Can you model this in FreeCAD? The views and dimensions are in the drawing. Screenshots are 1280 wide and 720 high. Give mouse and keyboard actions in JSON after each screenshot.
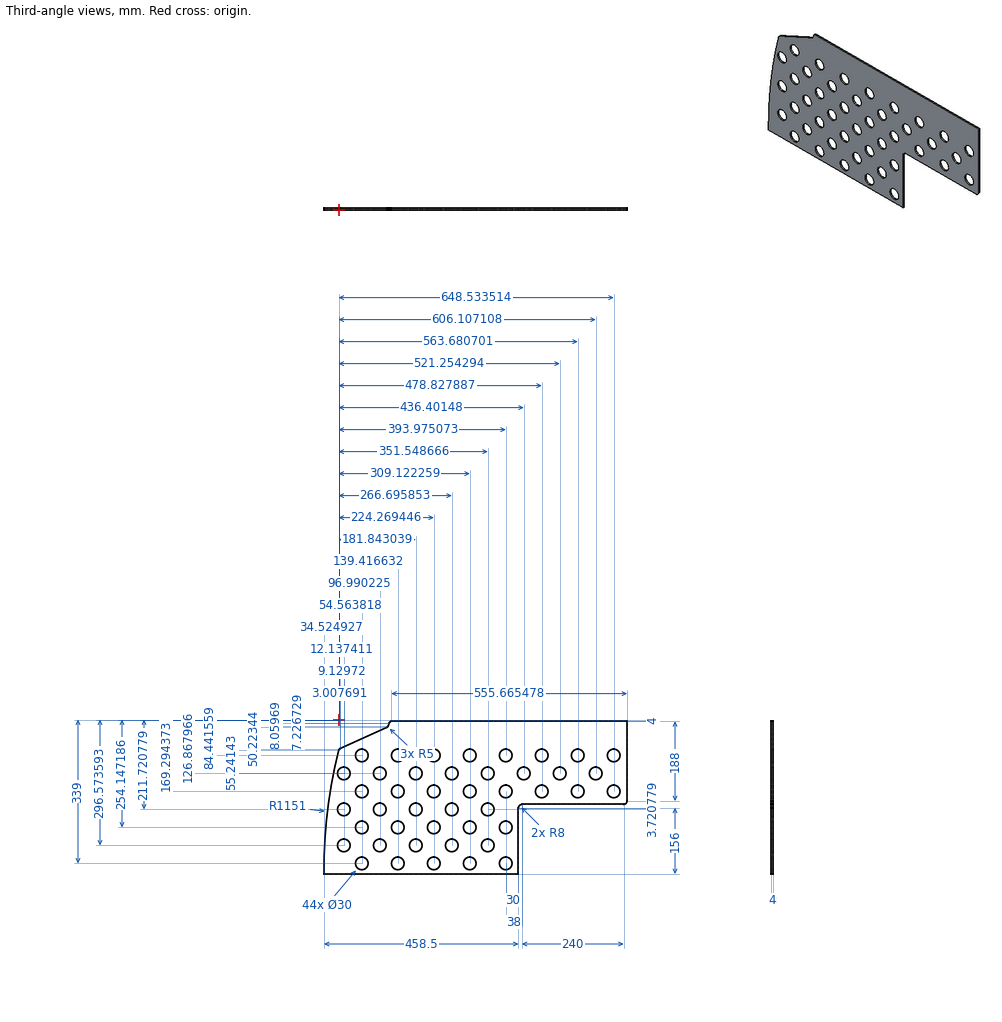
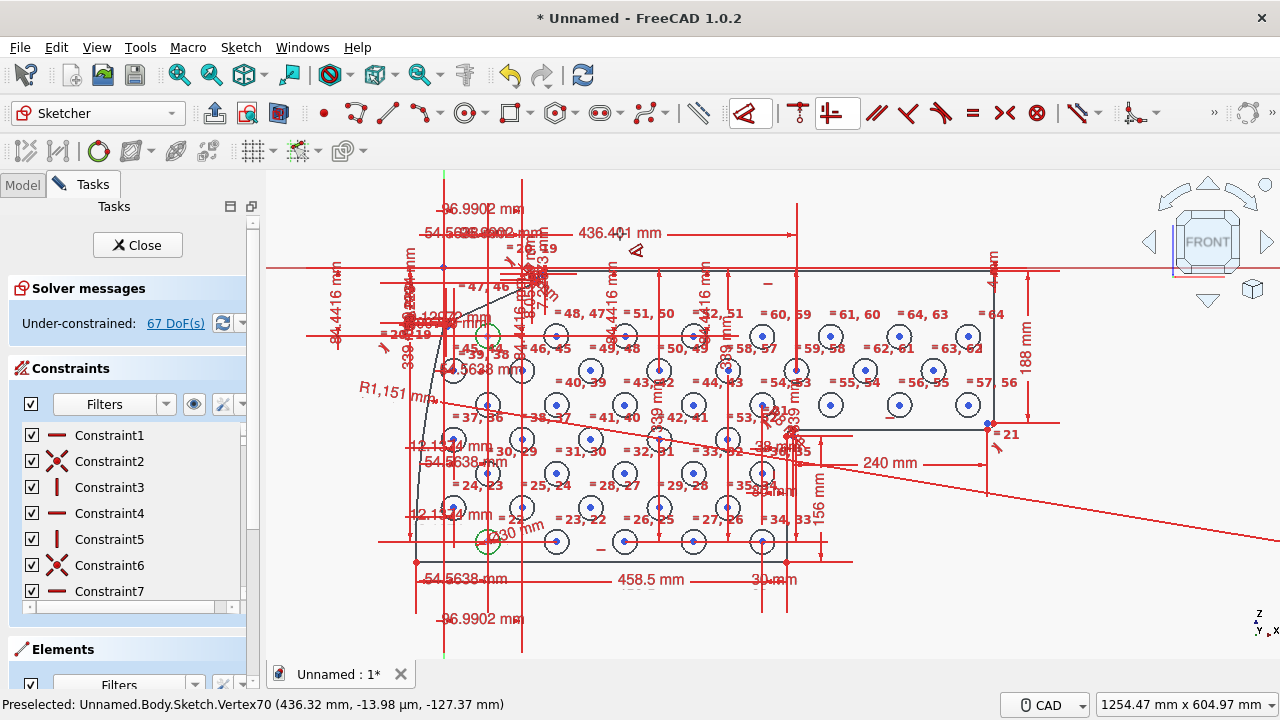
{"action": "left_click", "coordinate": [762, 337]}
{"action": "left_click", "coordinate": [796, 302]}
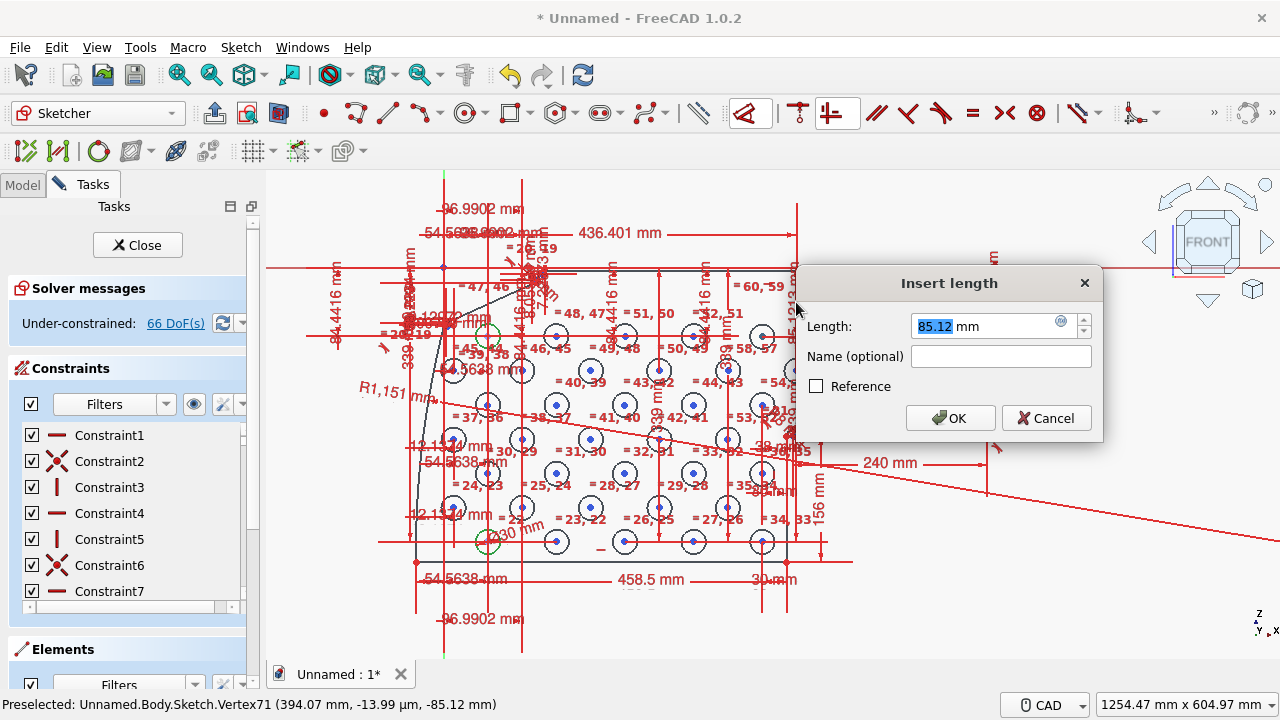
{"action": "type", "text": "84.441559"}
{"action": "key", "text": "Return"}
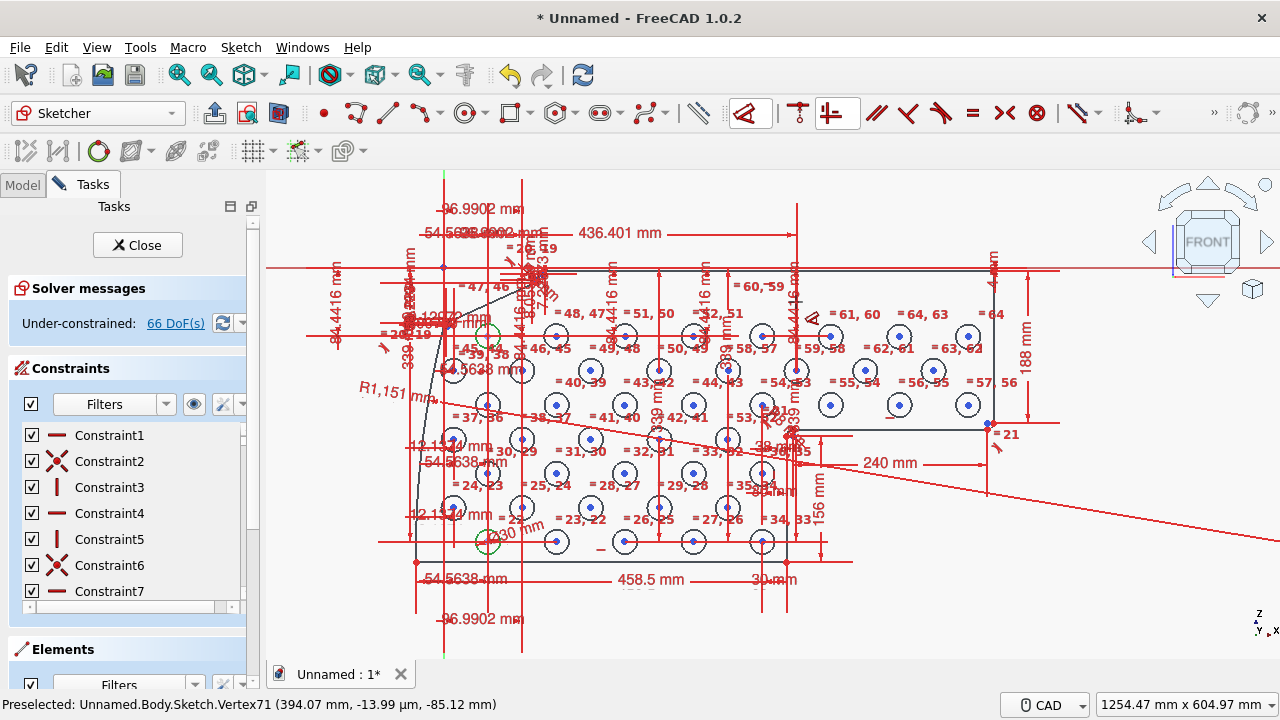
{"action": "left_click", "coordinate": [831, 337]}
{"action": "left_click", "coordinate": [865, 326]}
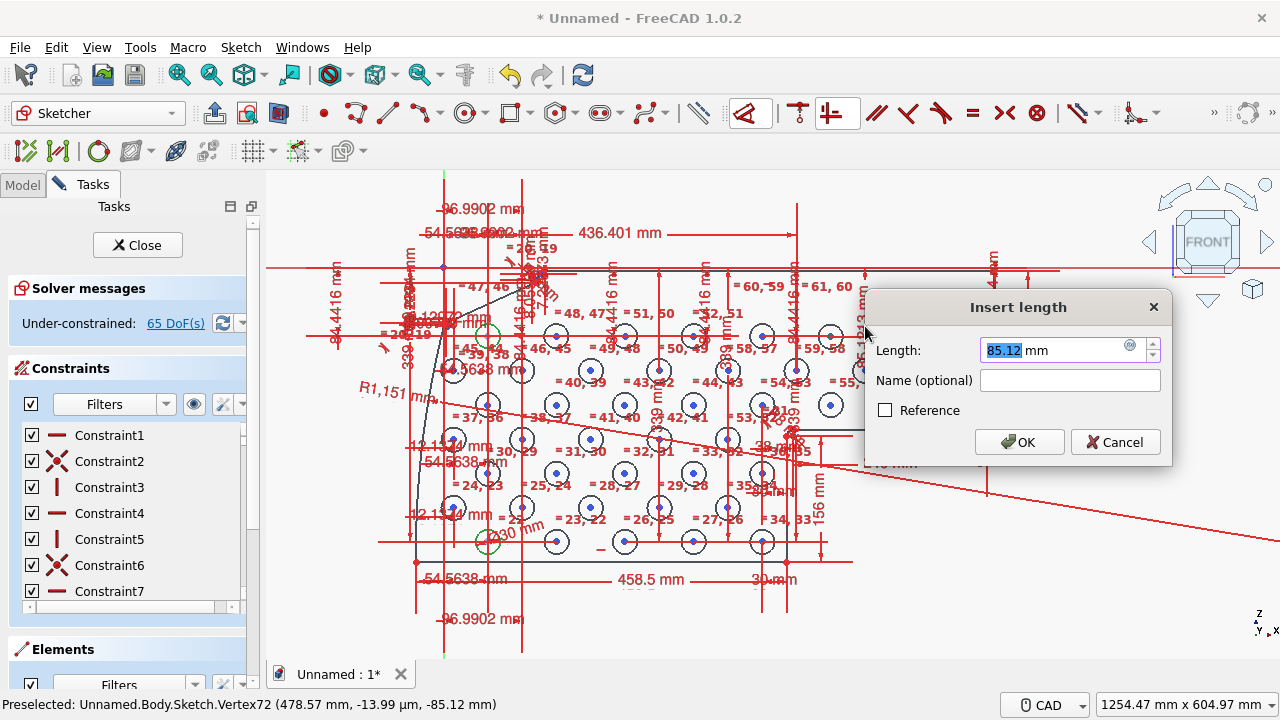
{"action": "type", "text": "84.441559"}
{"action": "key", "text": "Return"}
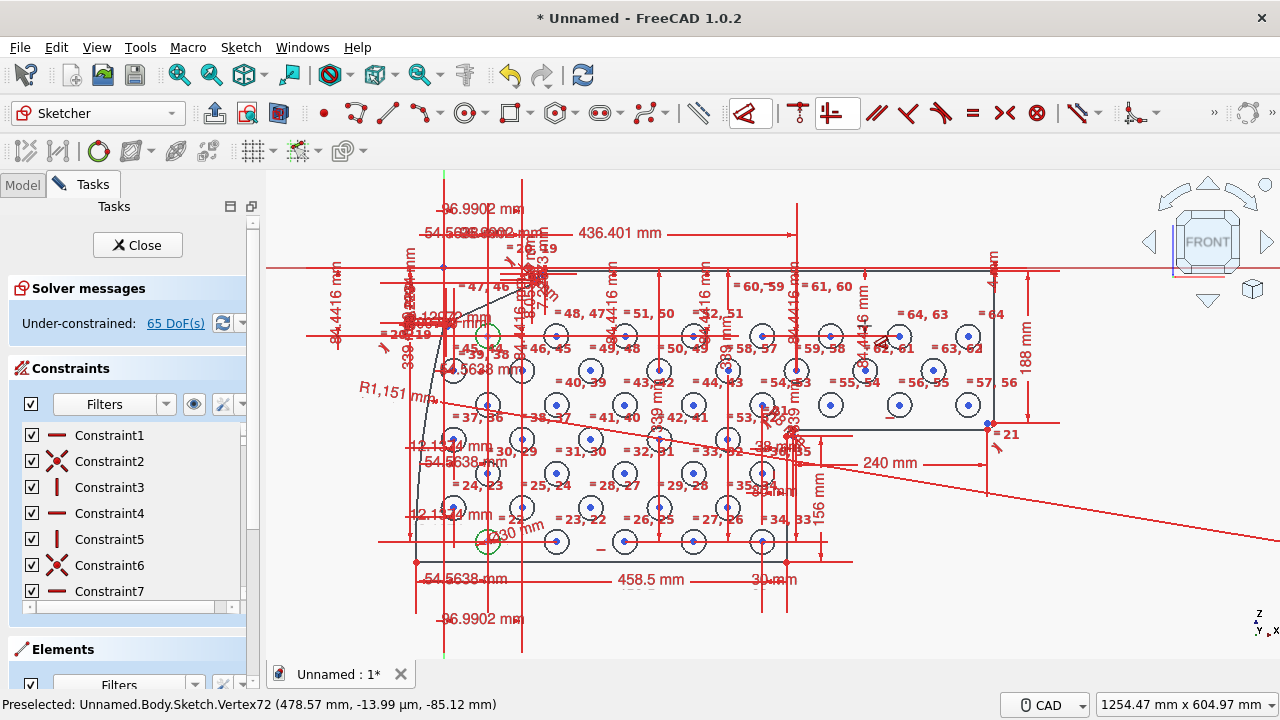
{"action": "left_click", "coordinate": [899, 337]}
{"action": "left_click", "coordinate": [933, 302]}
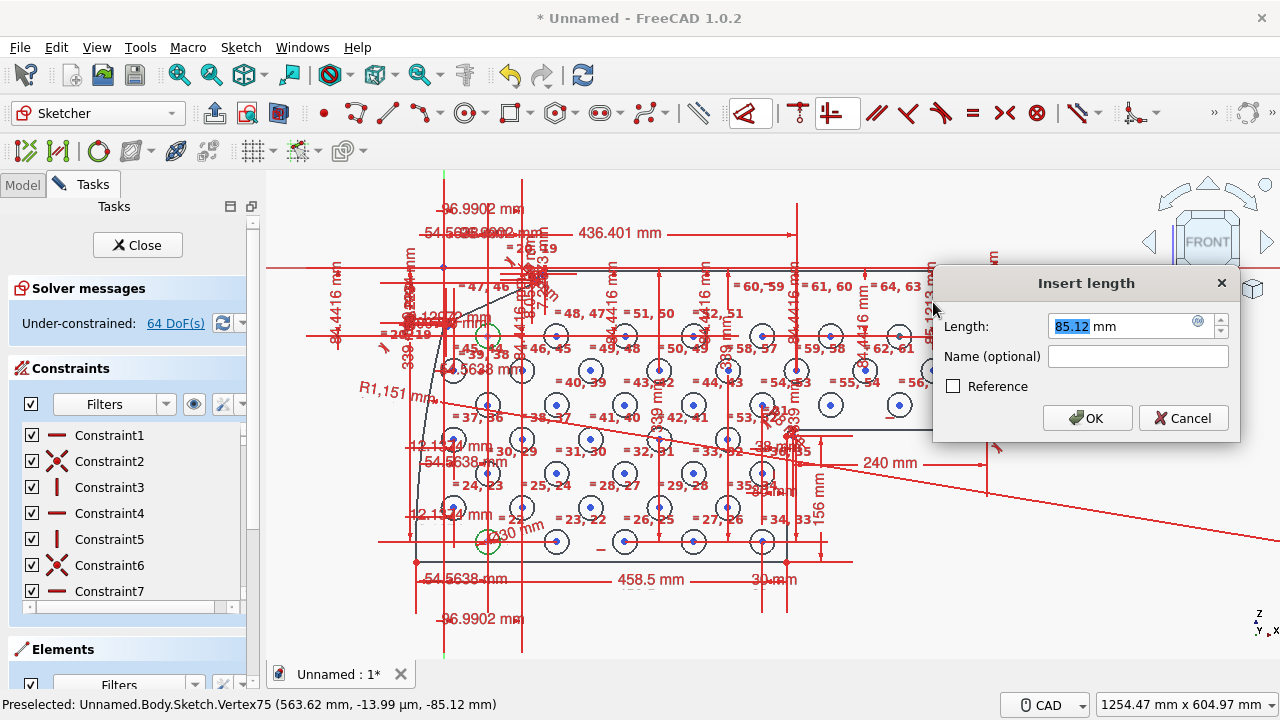
{"action": "type", "text": "84.441559"}
{"action": "key", "text": "Return"}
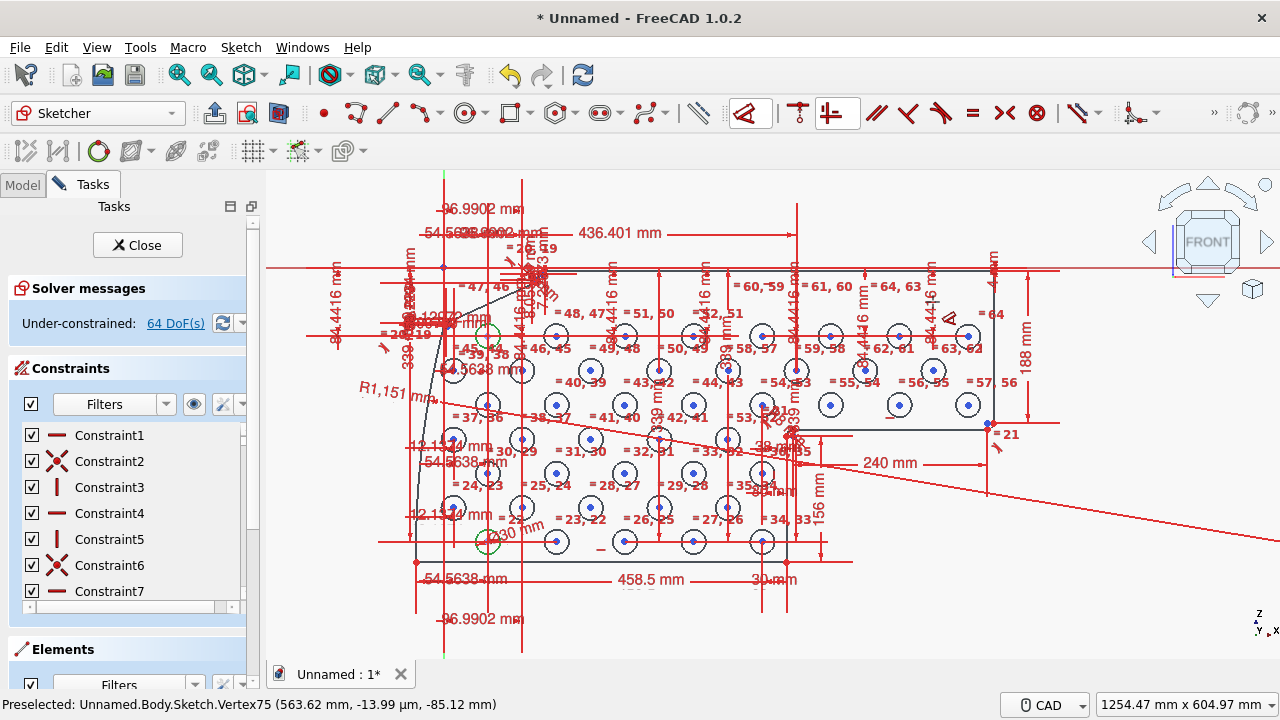
{"action": "left_click", "coordinate": [968, 337]}
{"action": "left_click", "coordinate": [1026, 302]}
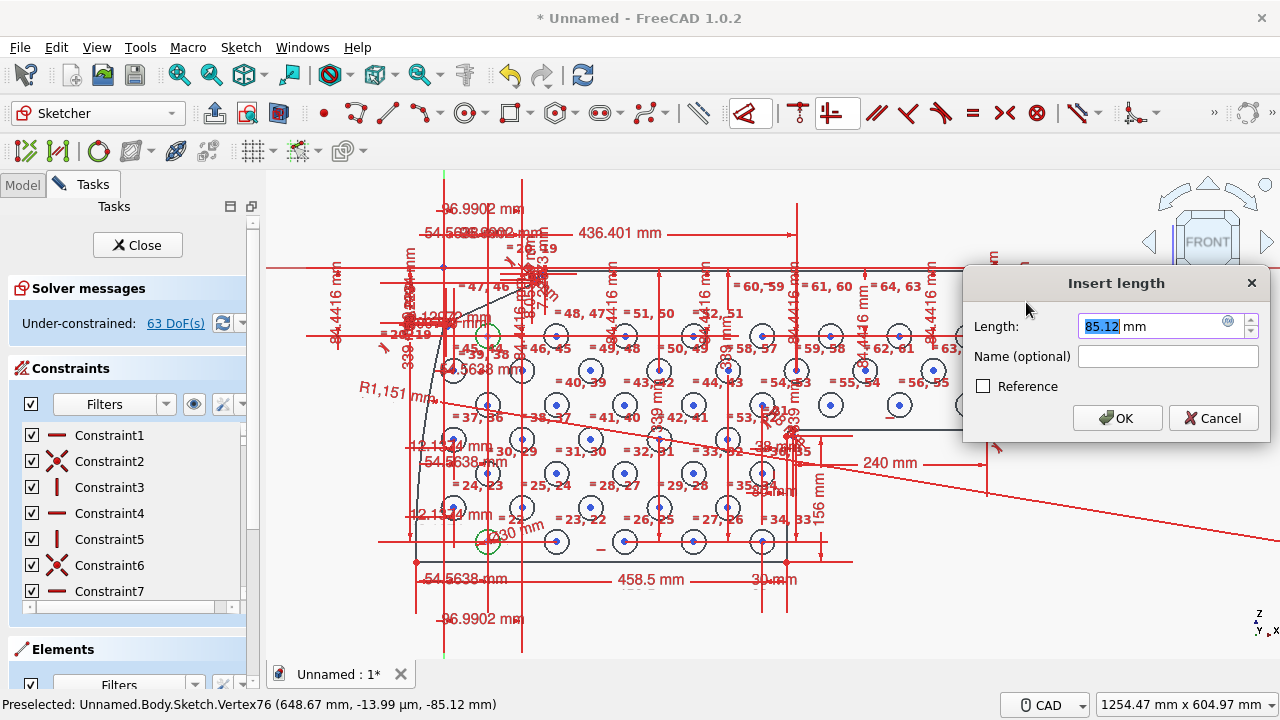
{"action": "type", "text": "84.441559"}
{"action": "key", "text": "Return"}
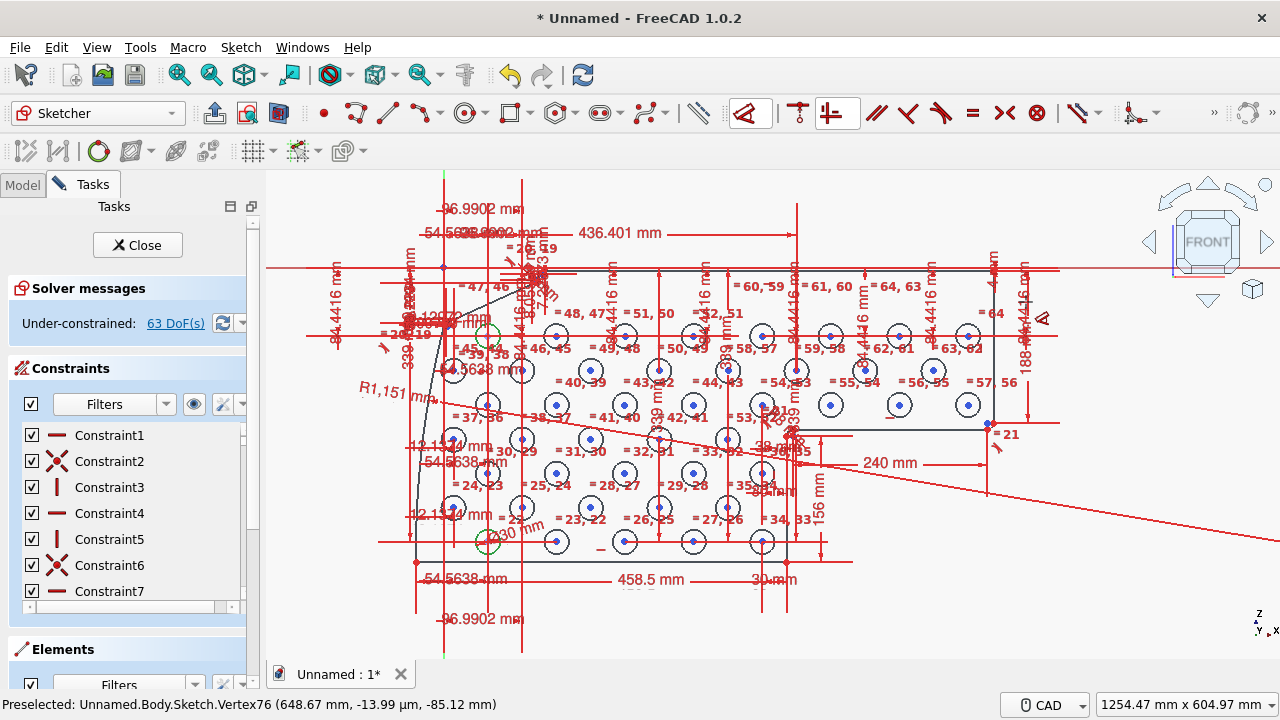
{"action": "scroll", "coordinate": [444, 326], "scroll_direction": "up", "scroll_amount": 7}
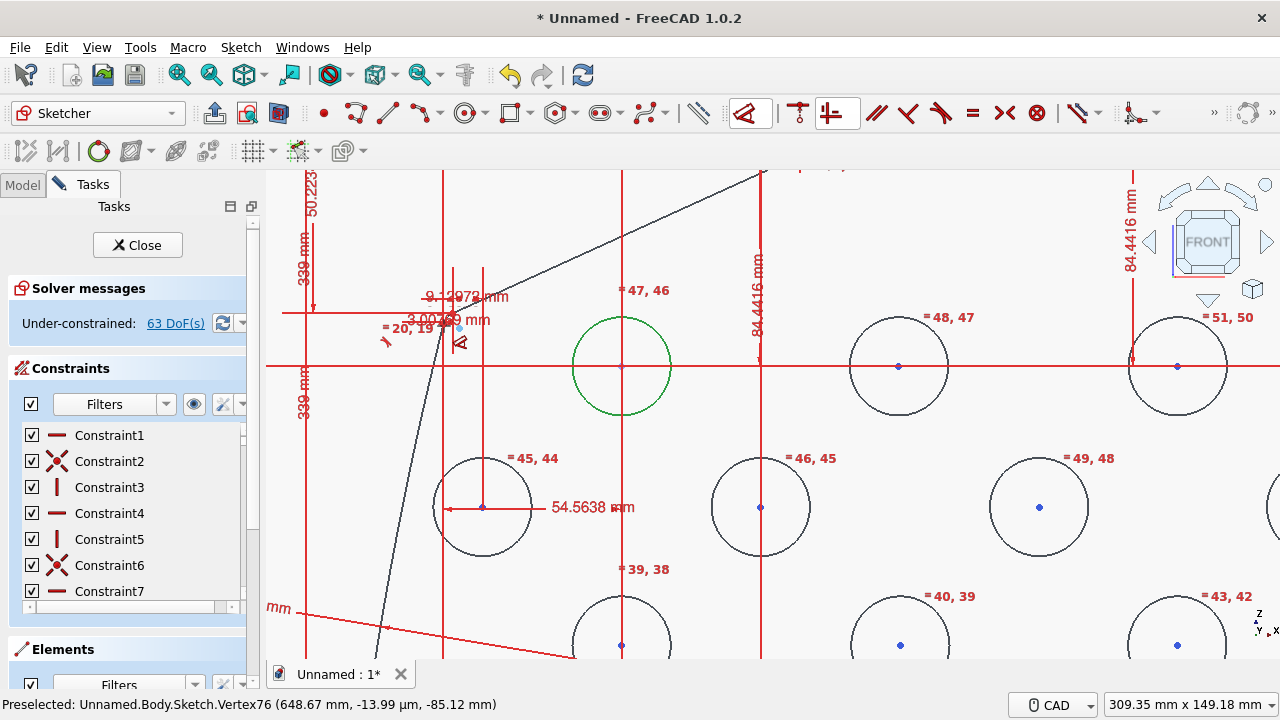
{"action": "left_click", "coordinate": [444, 324]}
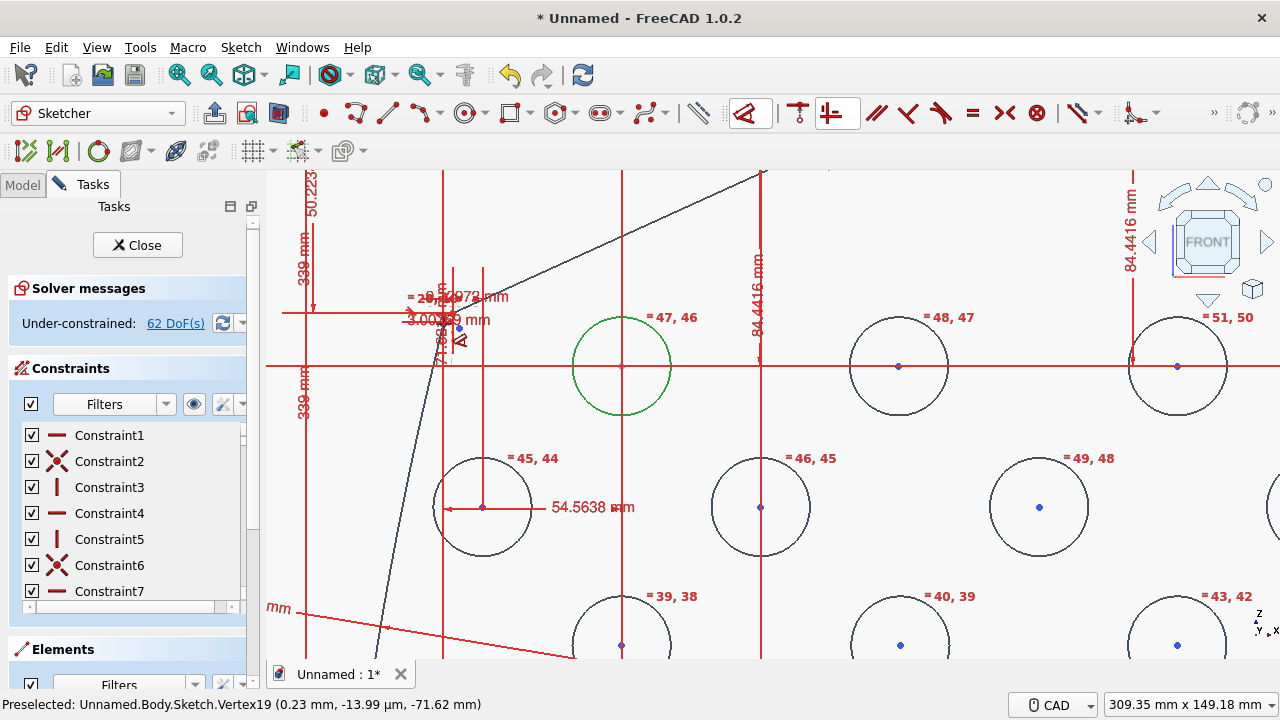
{"action": "scroll", "coordinate": [444, 326], "scroll_direction": "down", "scroll_amount": 7}